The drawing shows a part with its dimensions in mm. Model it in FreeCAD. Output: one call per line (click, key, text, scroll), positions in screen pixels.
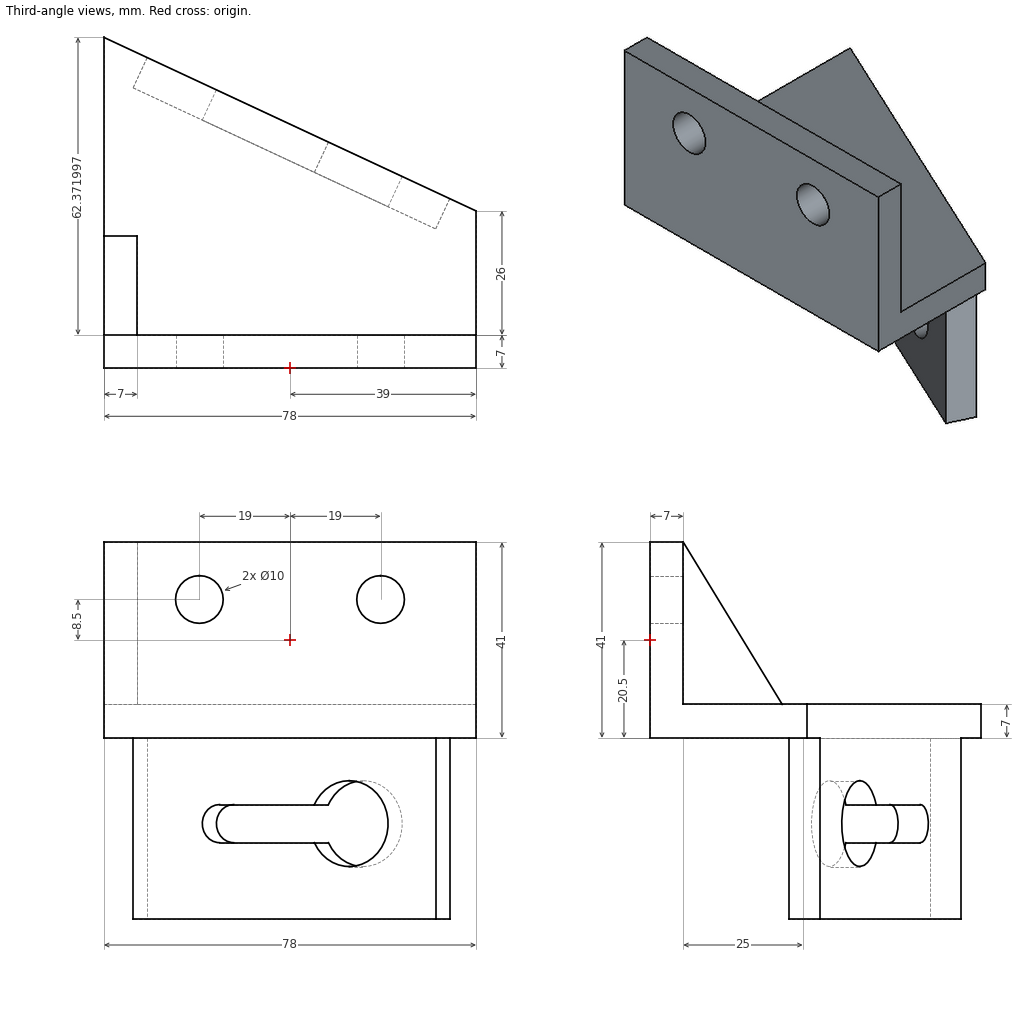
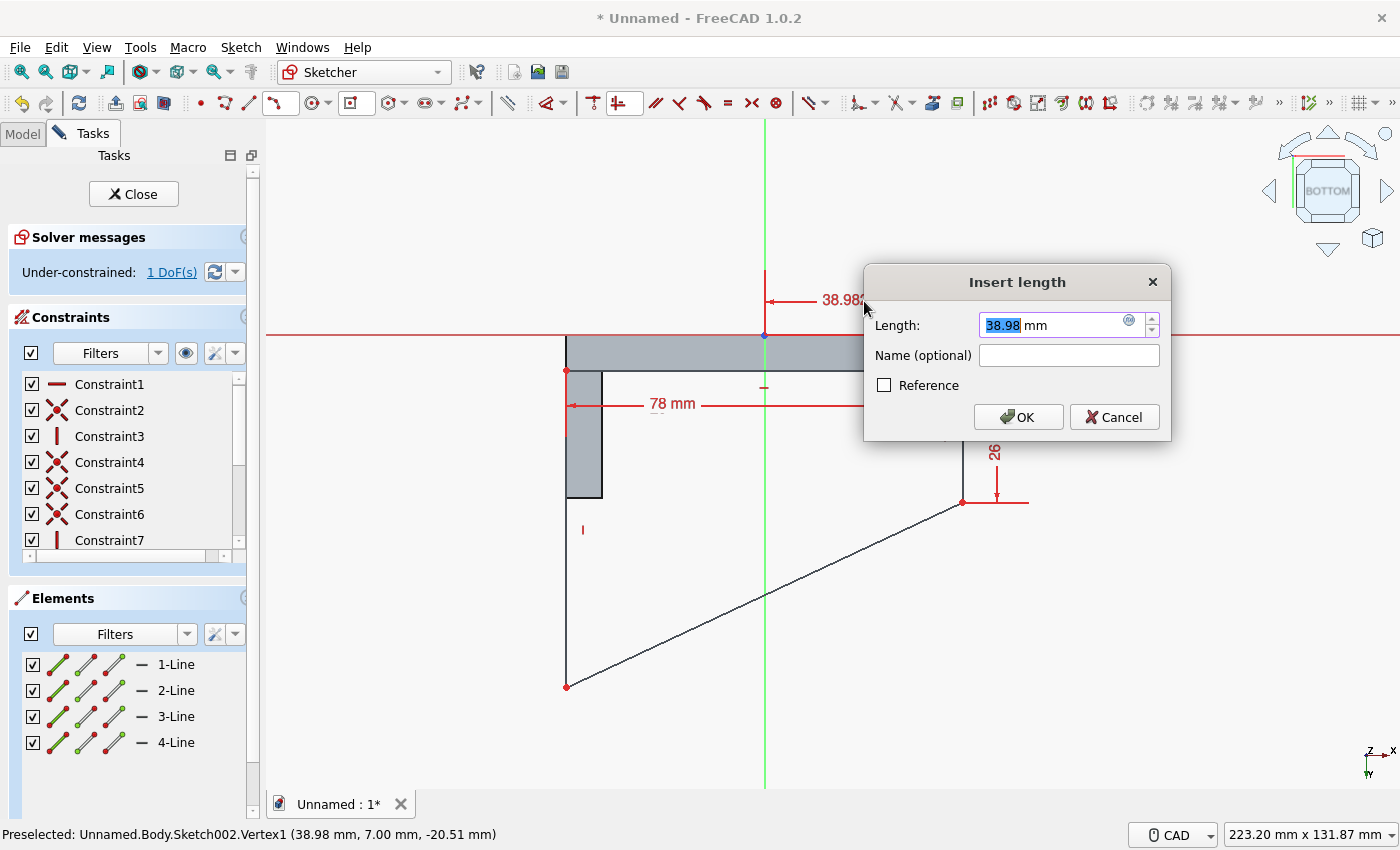
text(39)
key(Return)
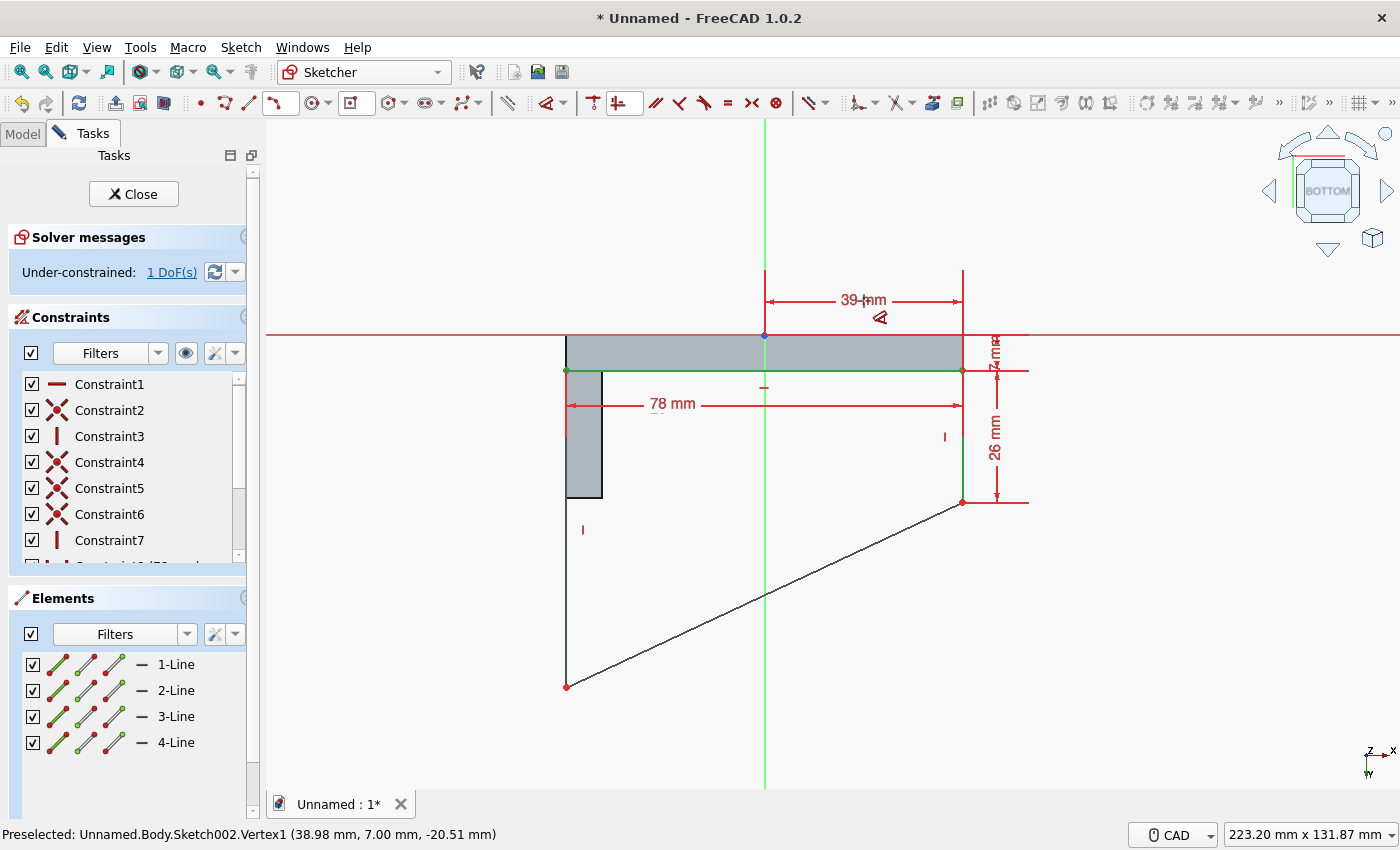
click(566, 466)
click(532, 529)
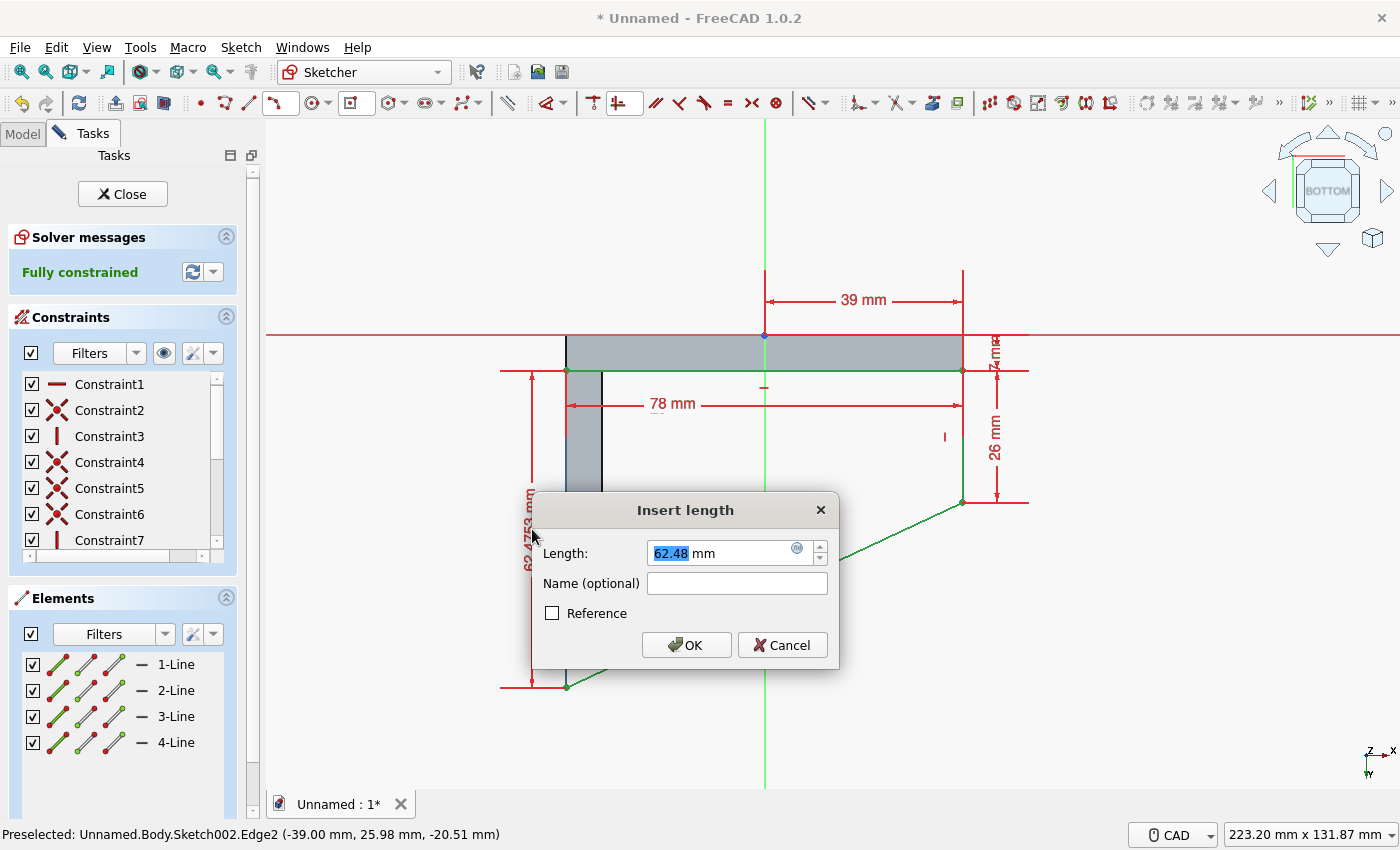
text(62.371997)
key(Return)
key(Escape)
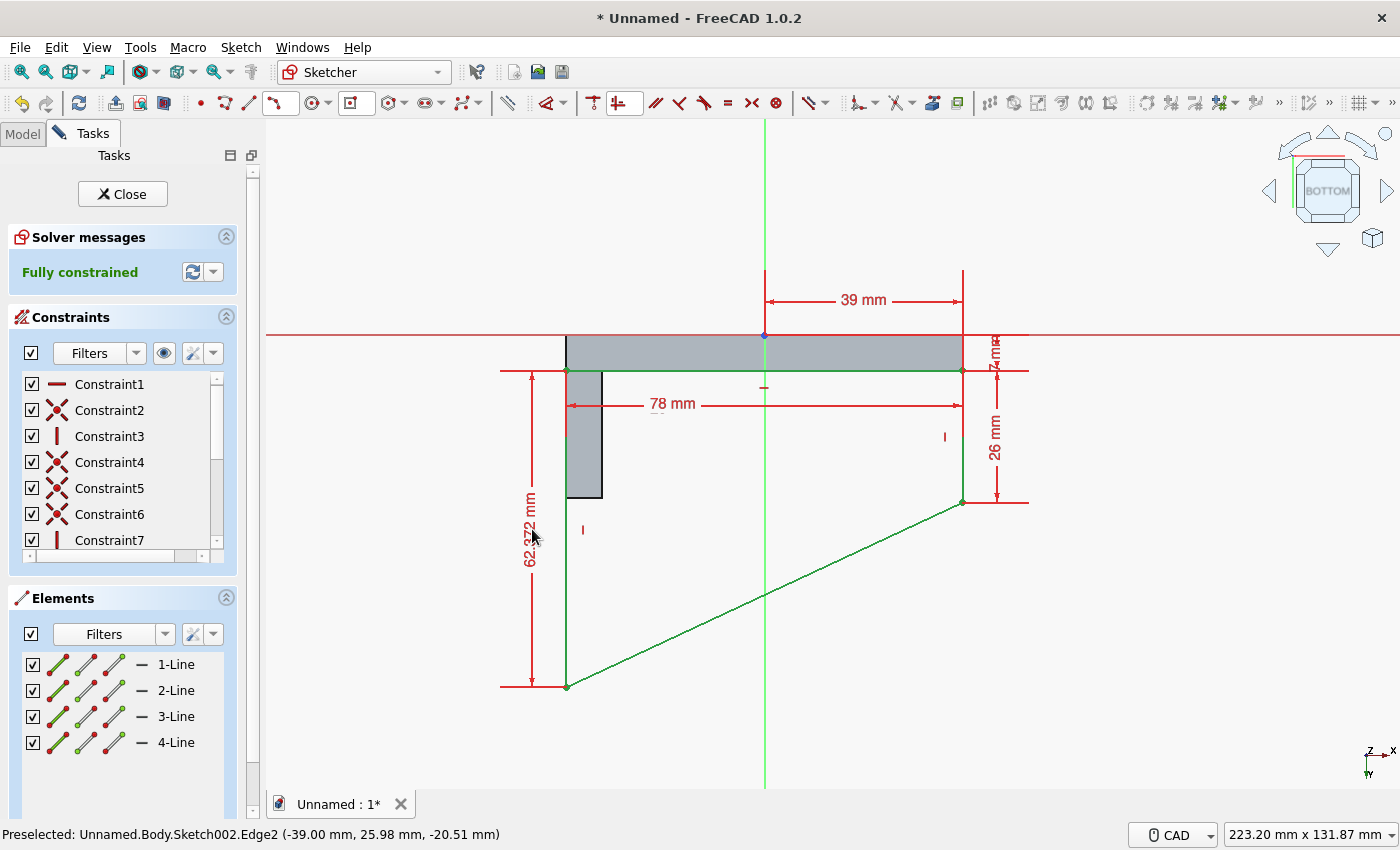
click(123, 194)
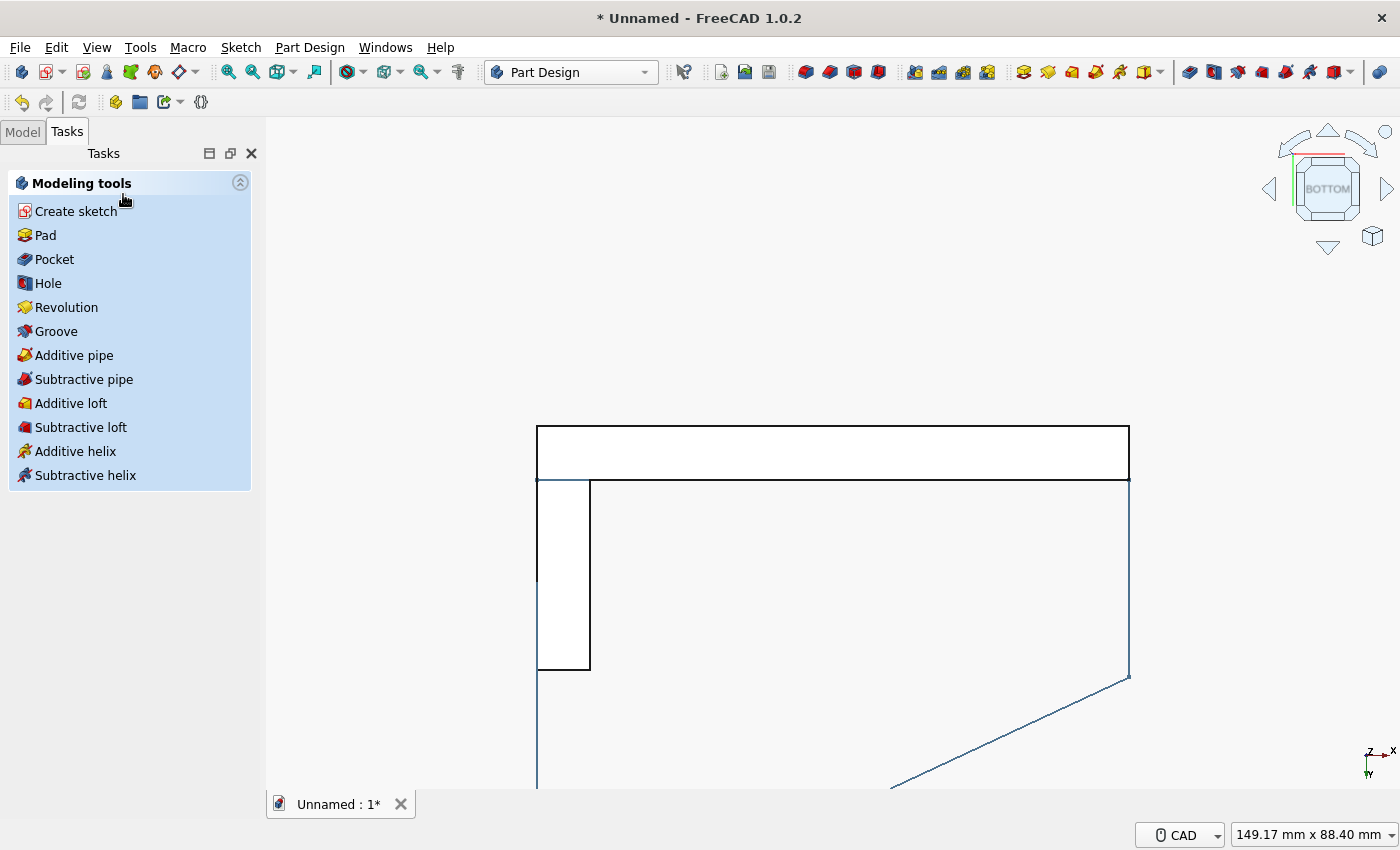
click(1024, 72)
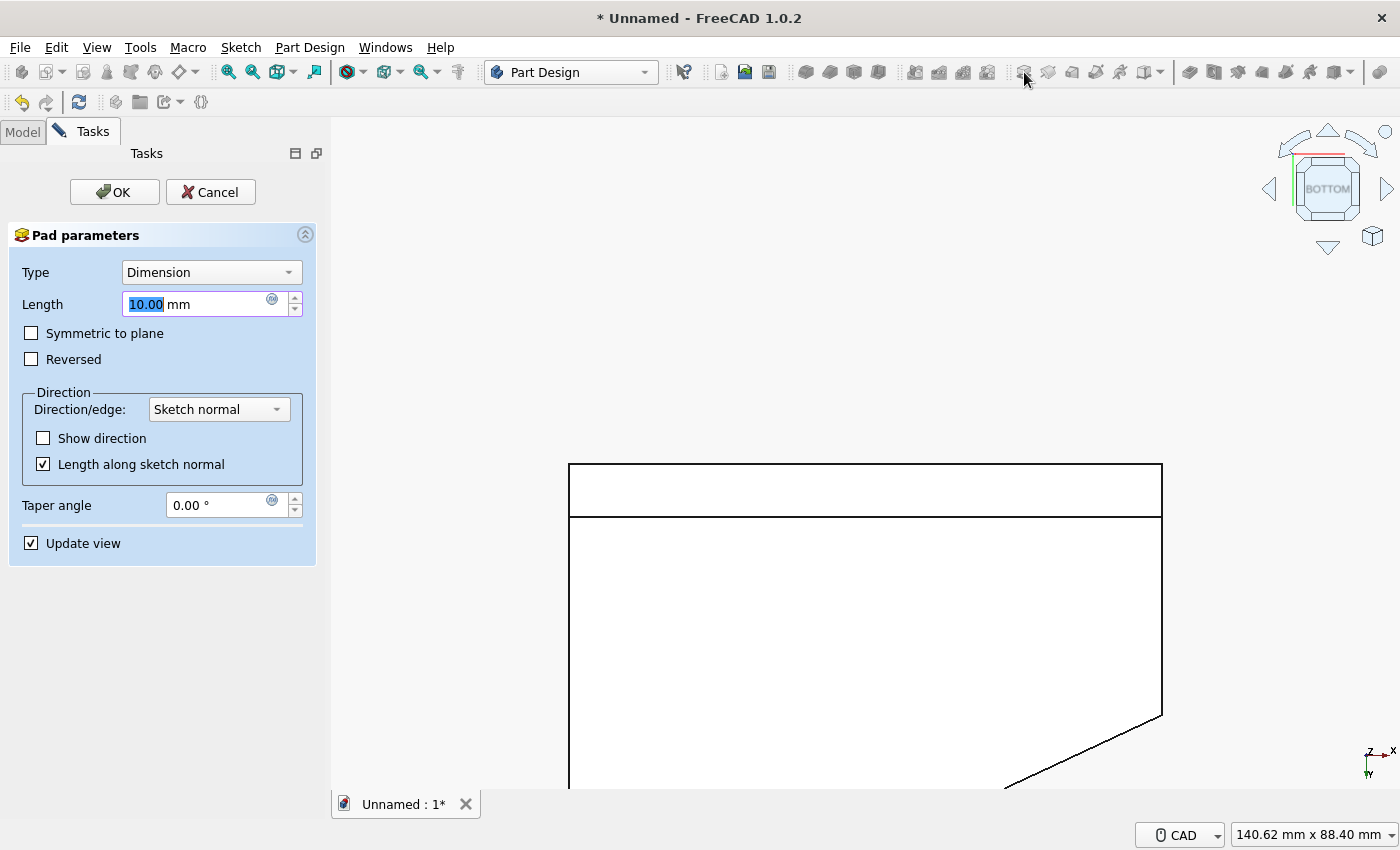
text(7)
key(Tab)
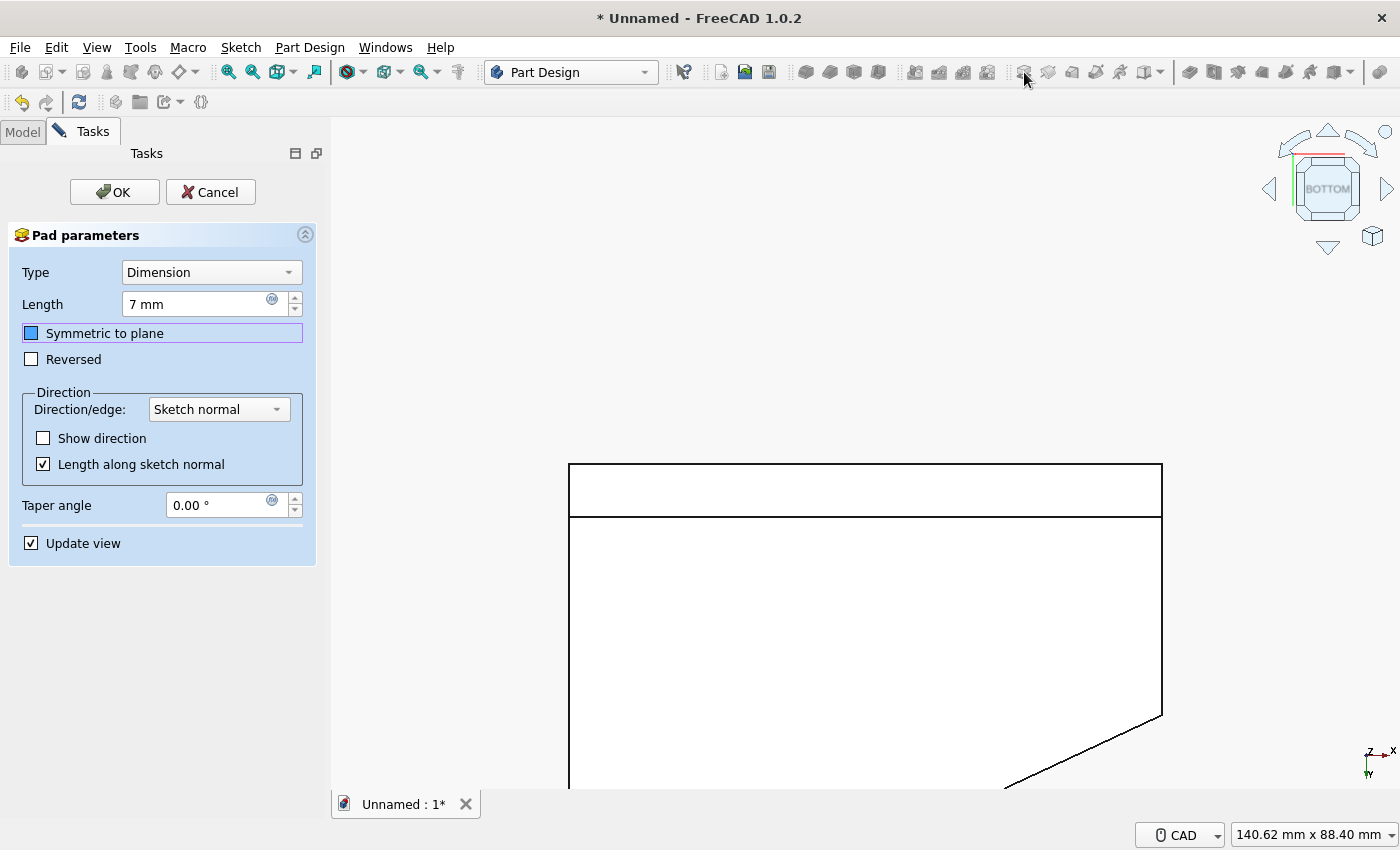
click(30, 359)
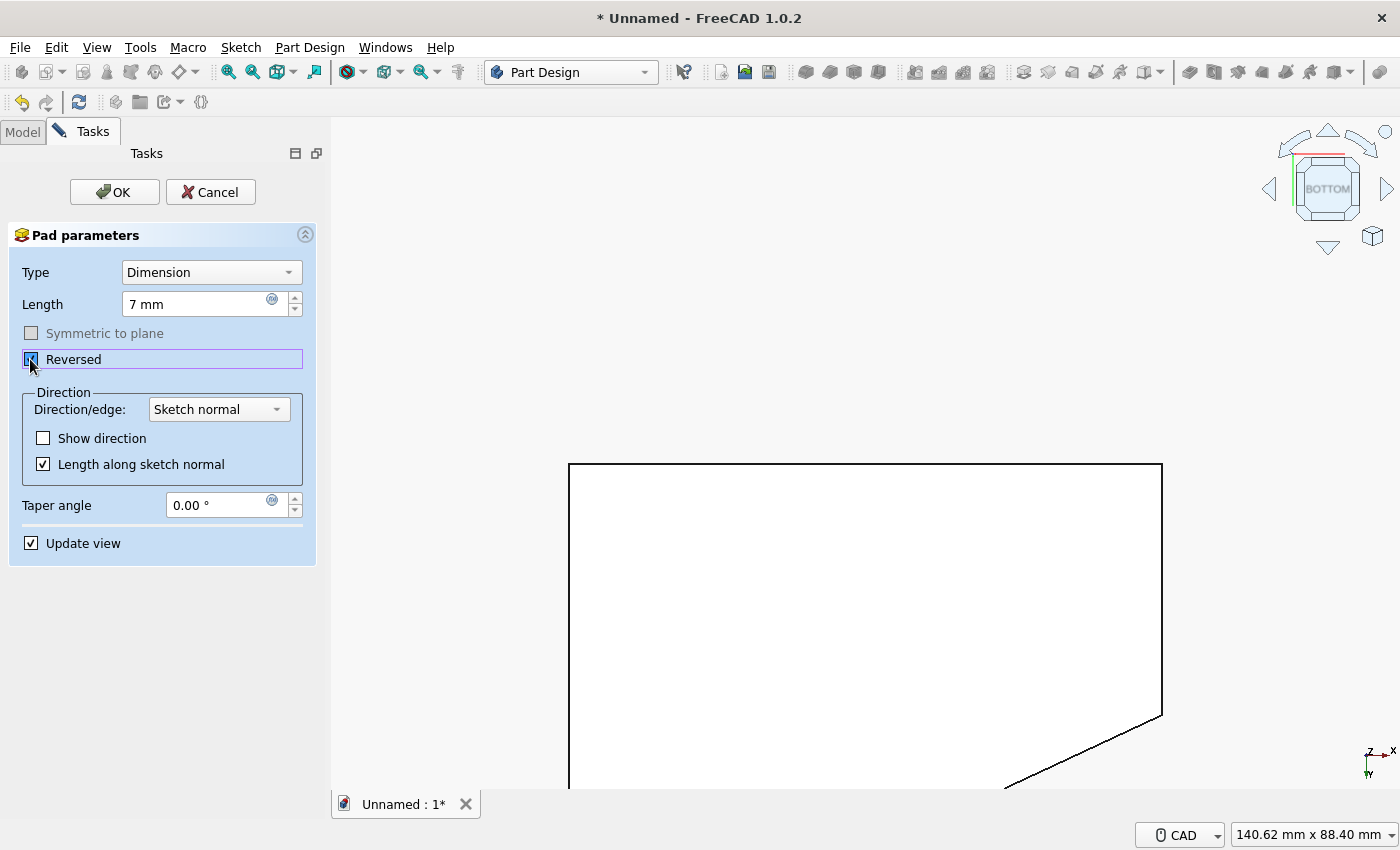
click(115, 192)